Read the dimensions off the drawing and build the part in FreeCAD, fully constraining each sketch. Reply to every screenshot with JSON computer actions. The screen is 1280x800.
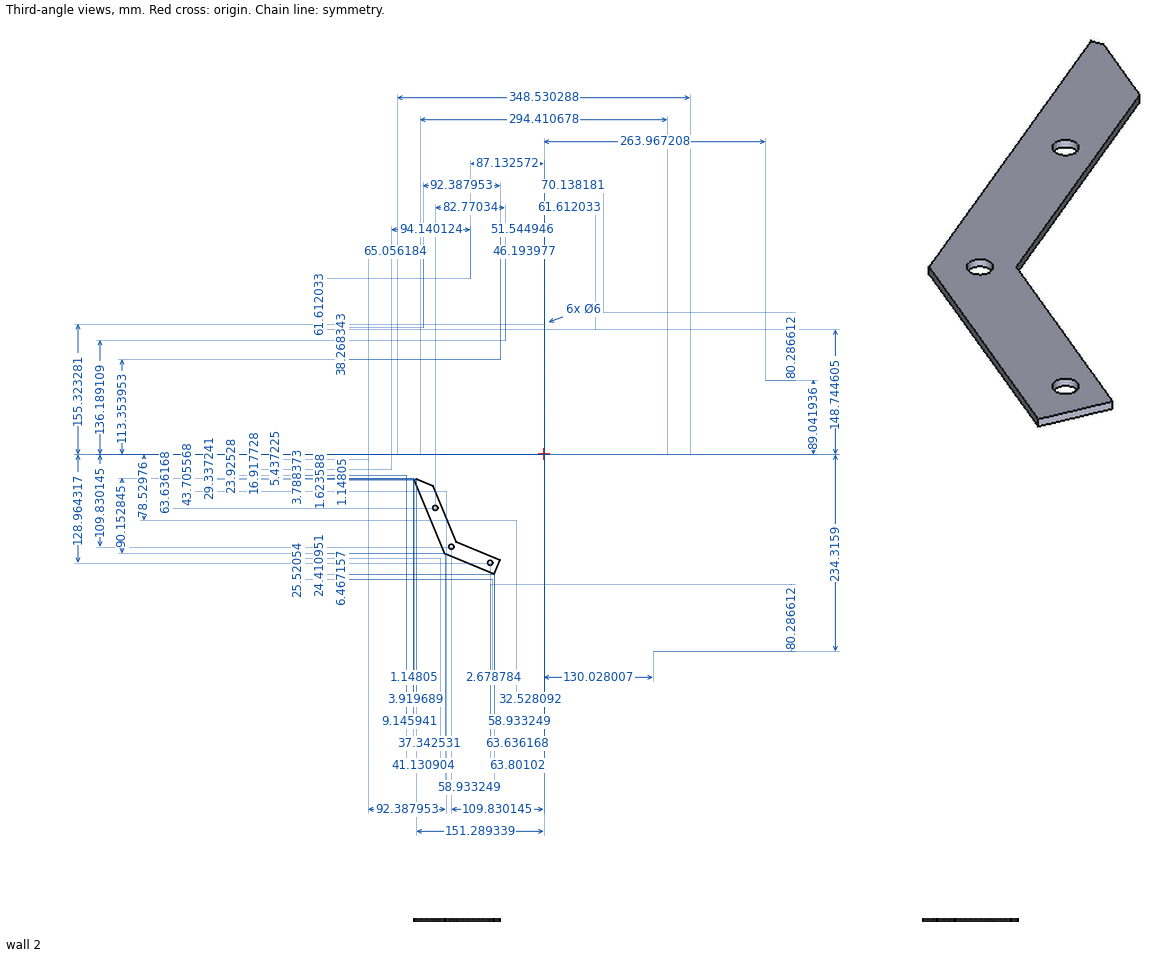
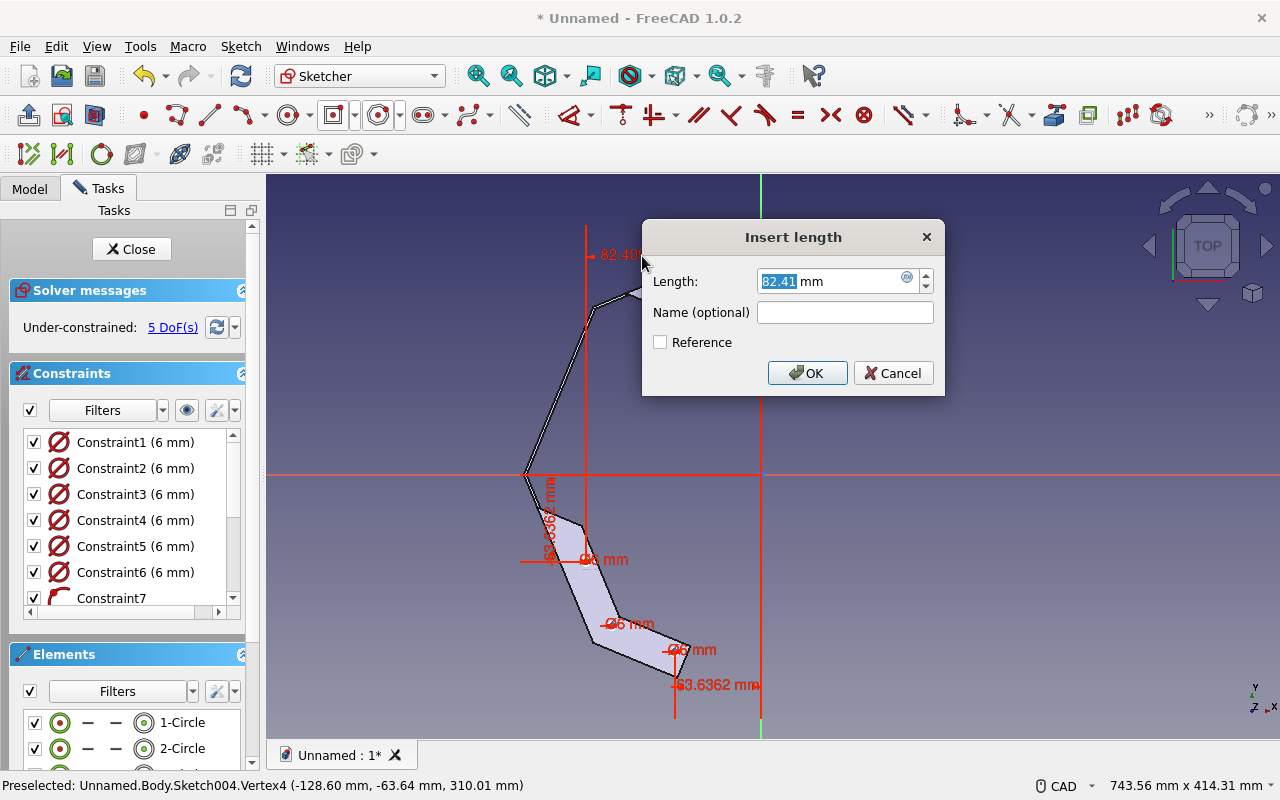
{"action": "type", "text": "82.77034"}
{"action": "key", "text": "Return"}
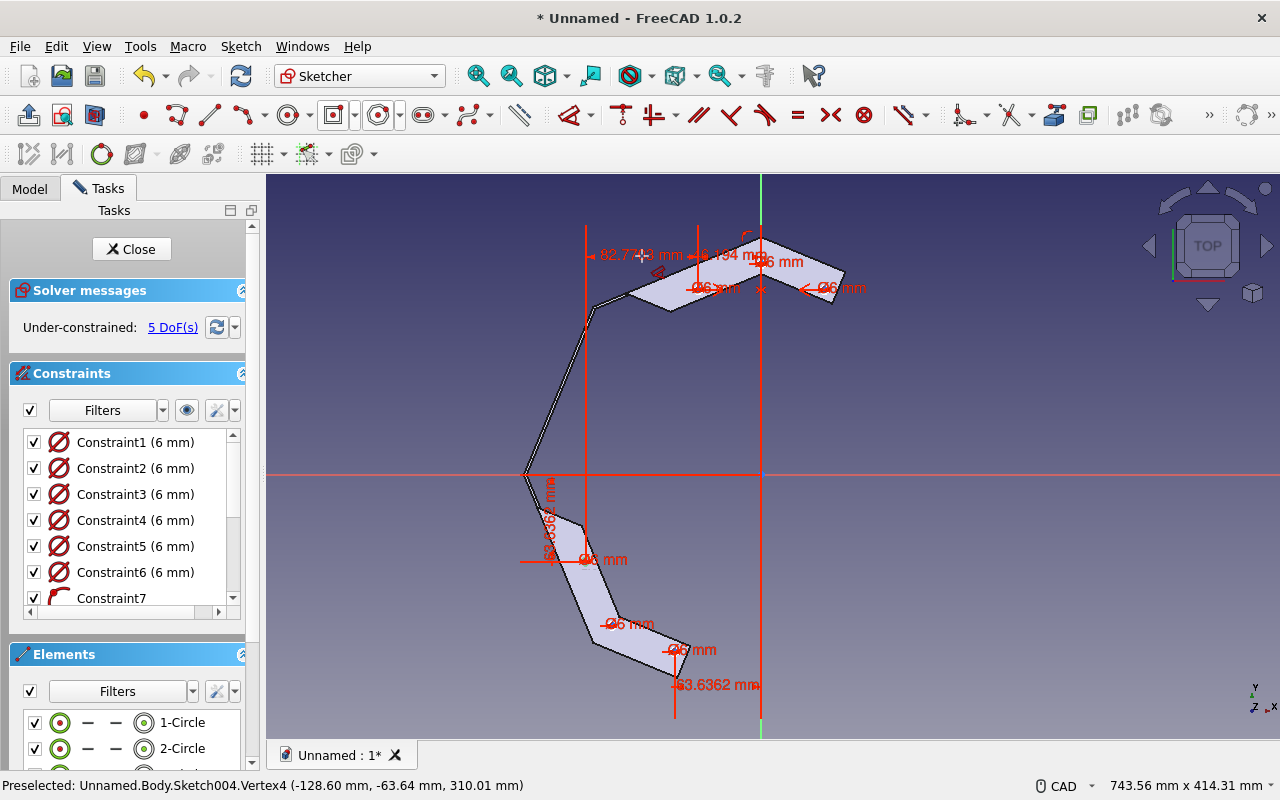
{"action": "left_click", "coordinate": [761, 264]}
{"action": "left_click", "coordinate": [795, 369]}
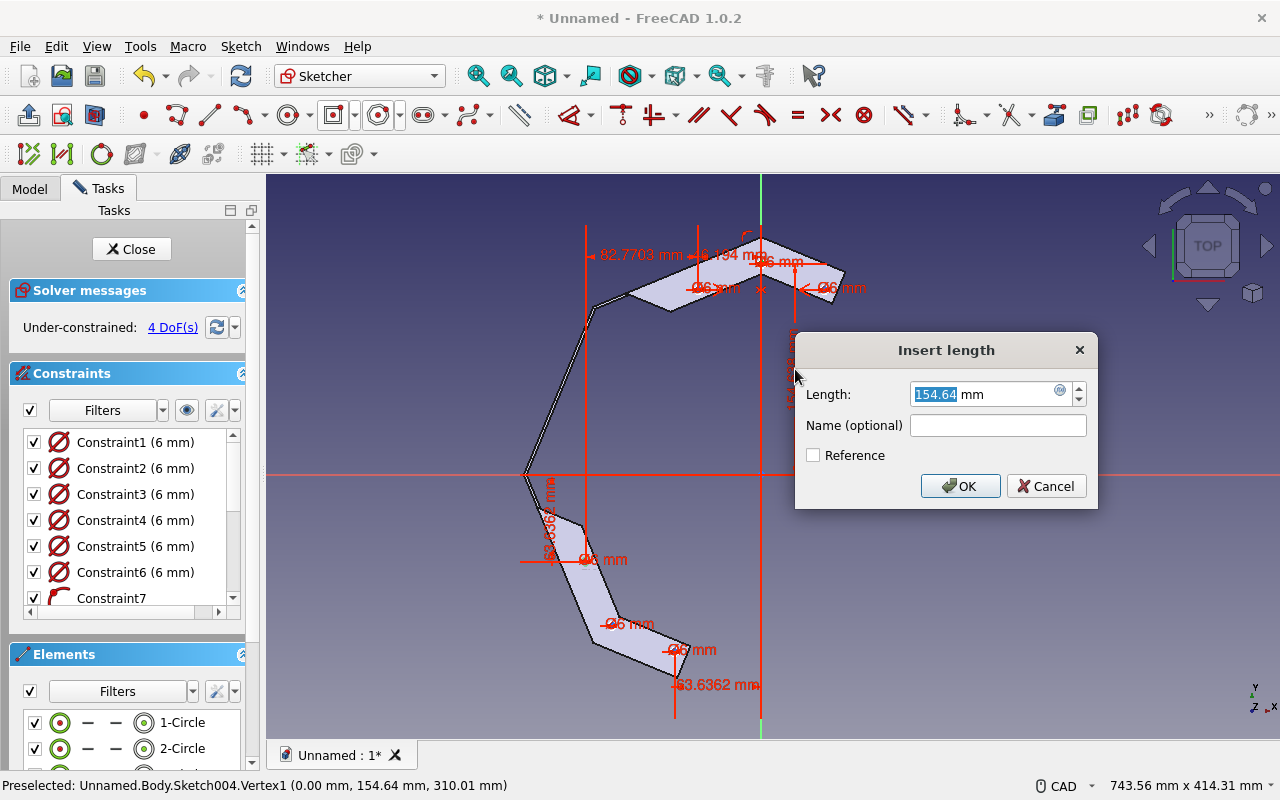
{"action": "type", "text": "155.323281"}
{"action": "key", "text": "Return"}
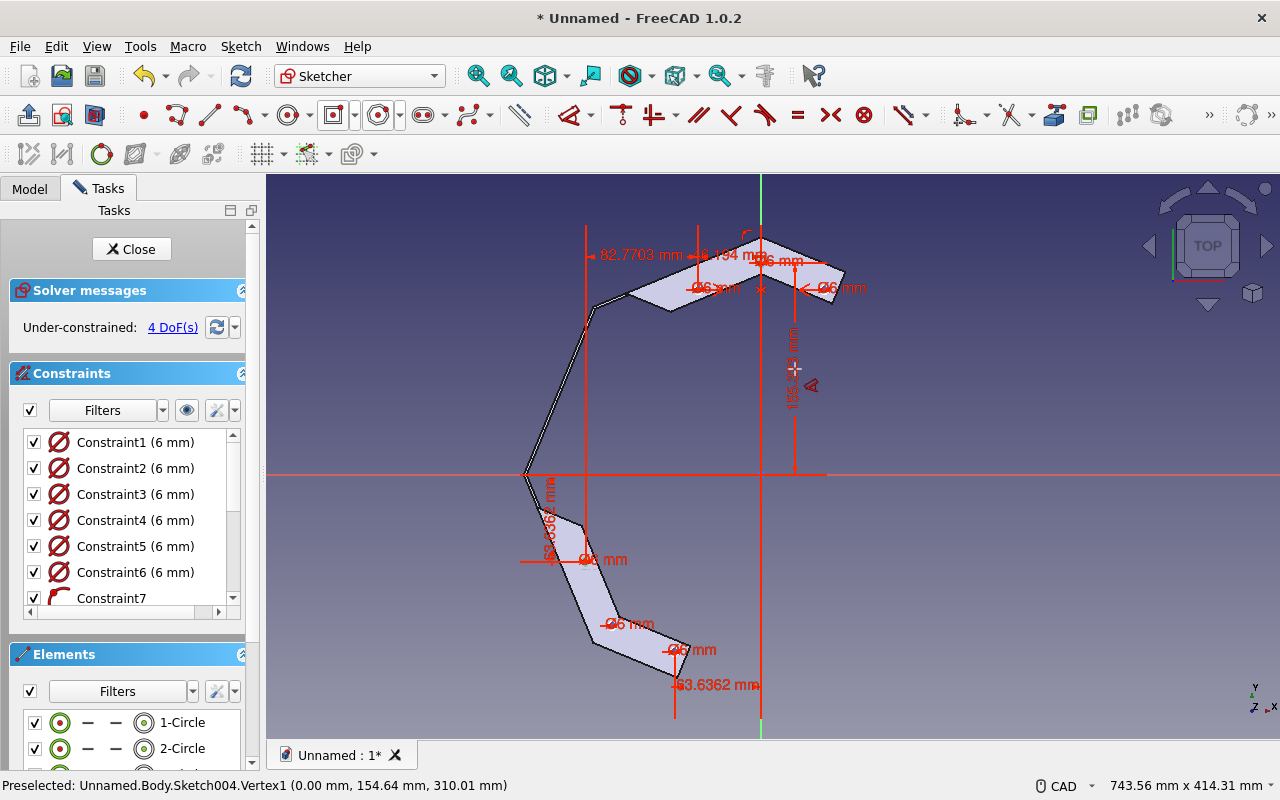
{"action": "left_click", "coordinate": [698, 290]}
{"action": "left_click", "coordinate": [795, 340]}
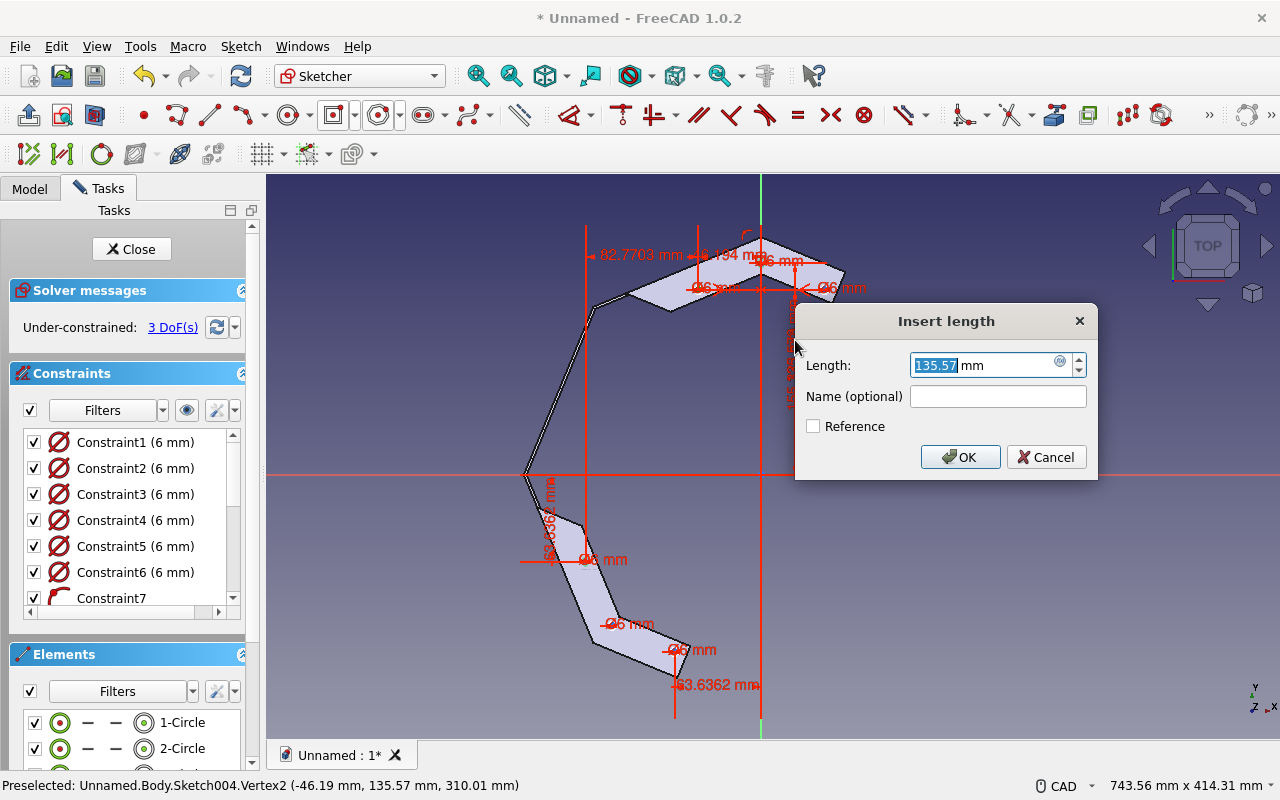
{"action": "type", "text": "136.189109"}
{"action": "key", "text": "Return"}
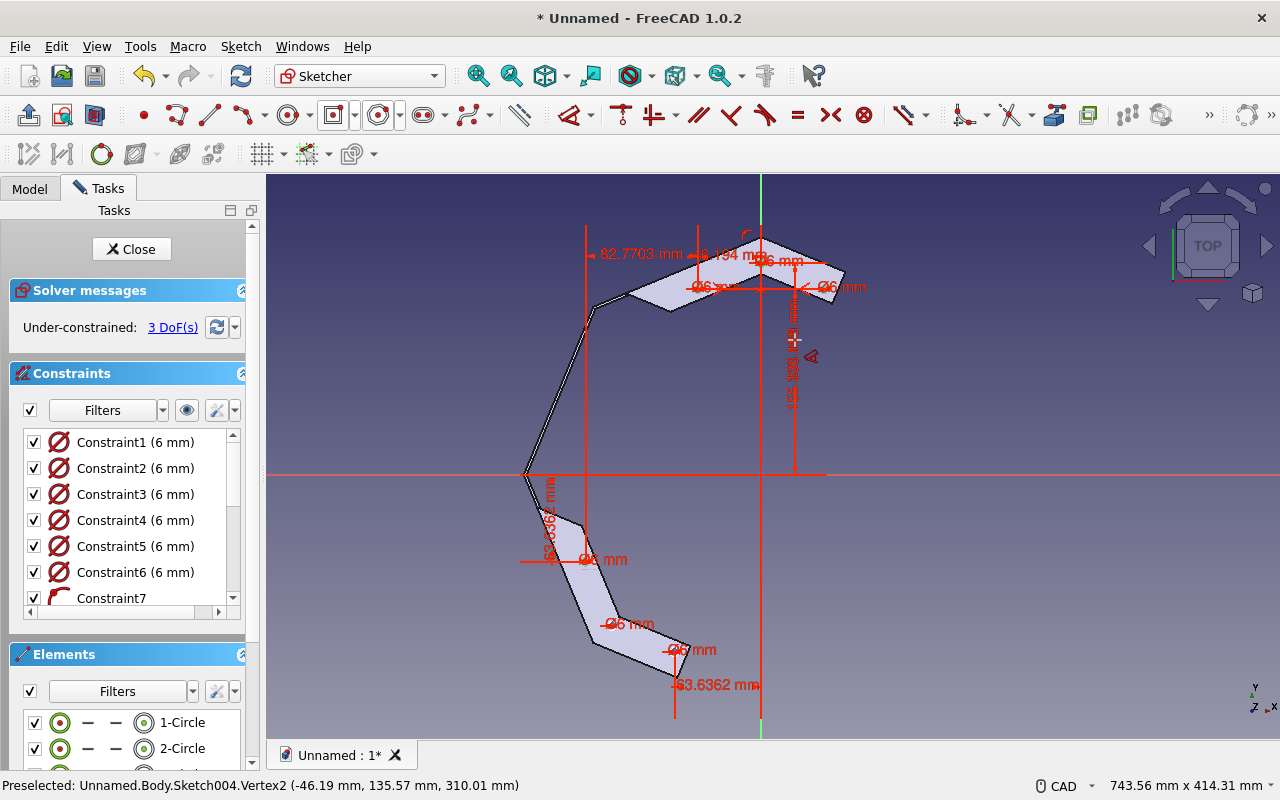
{"action": "left_click", "coordinate": [610, 628]}
{"action": "left_click", "coordinate": [652, 660]}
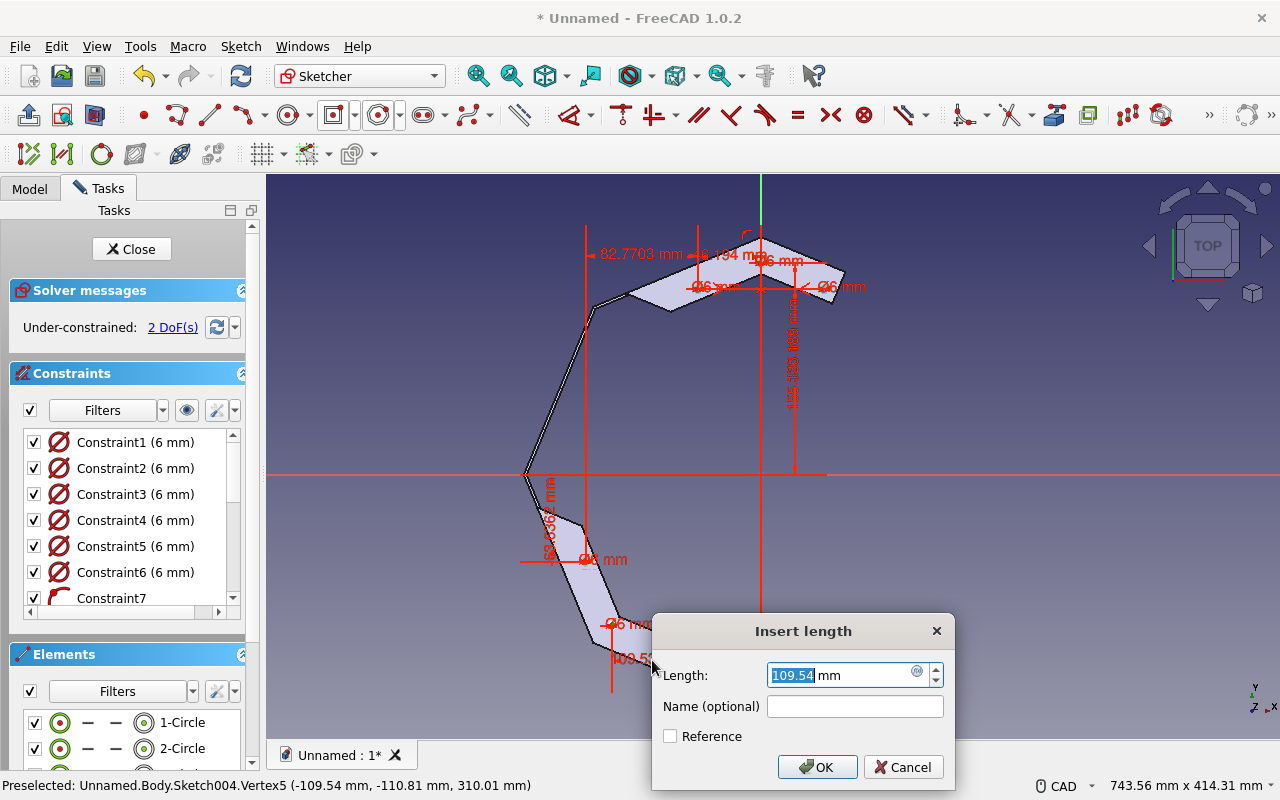
{"action": "type", "text": "109.830145"}
{"action": "key", "text": "Return"}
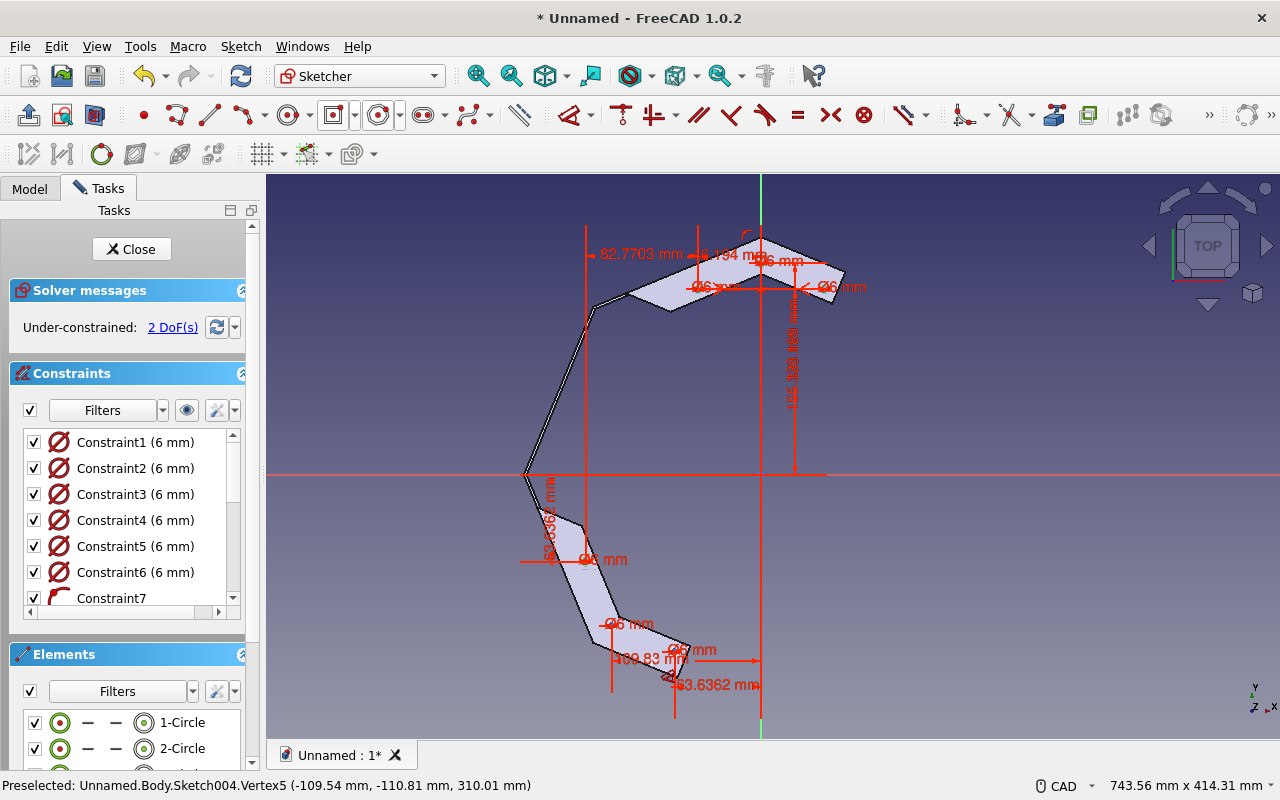
{"action": "left_click", "coordinate": [612, 626]}
{"action": "left_click", "coordinate": [578, 585]}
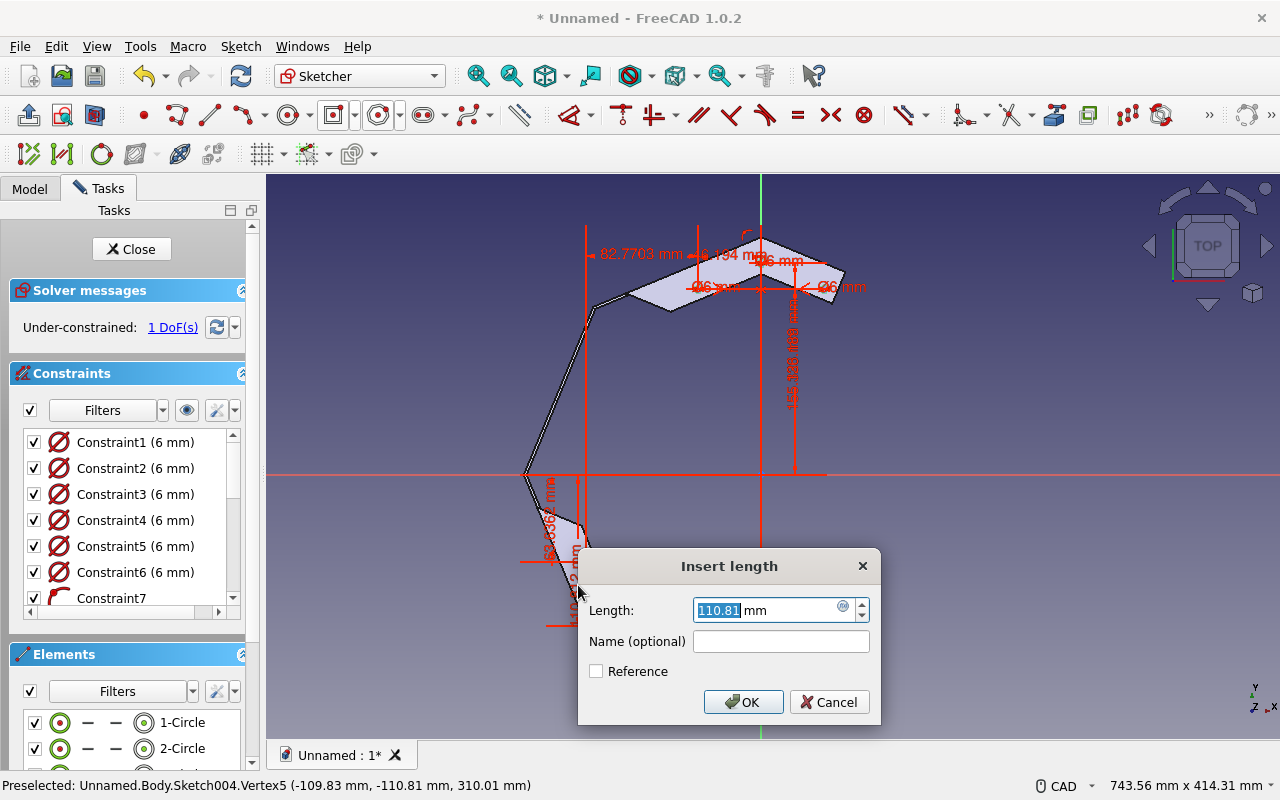
{"action": "type", "text": "109.830145"}
{"action": "key", "text": "Return"}